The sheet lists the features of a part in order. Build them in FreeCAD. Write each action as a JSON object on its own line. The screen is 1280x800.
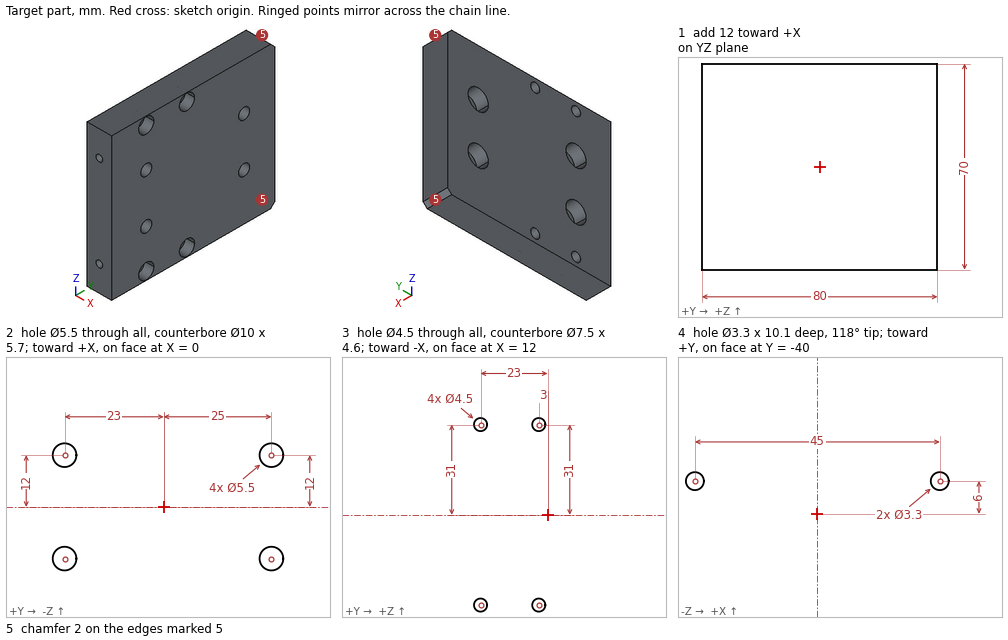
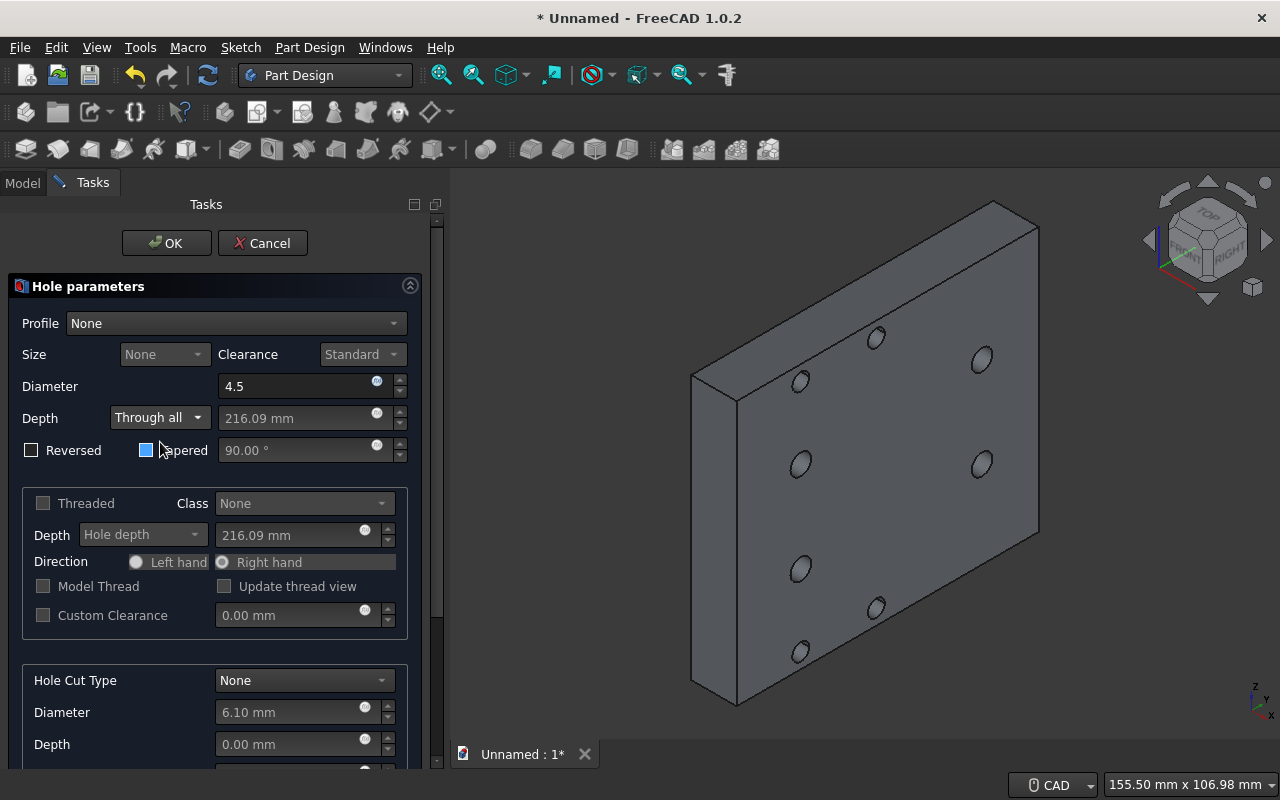
{"action": "left_click", "coordinate": [306, 680]}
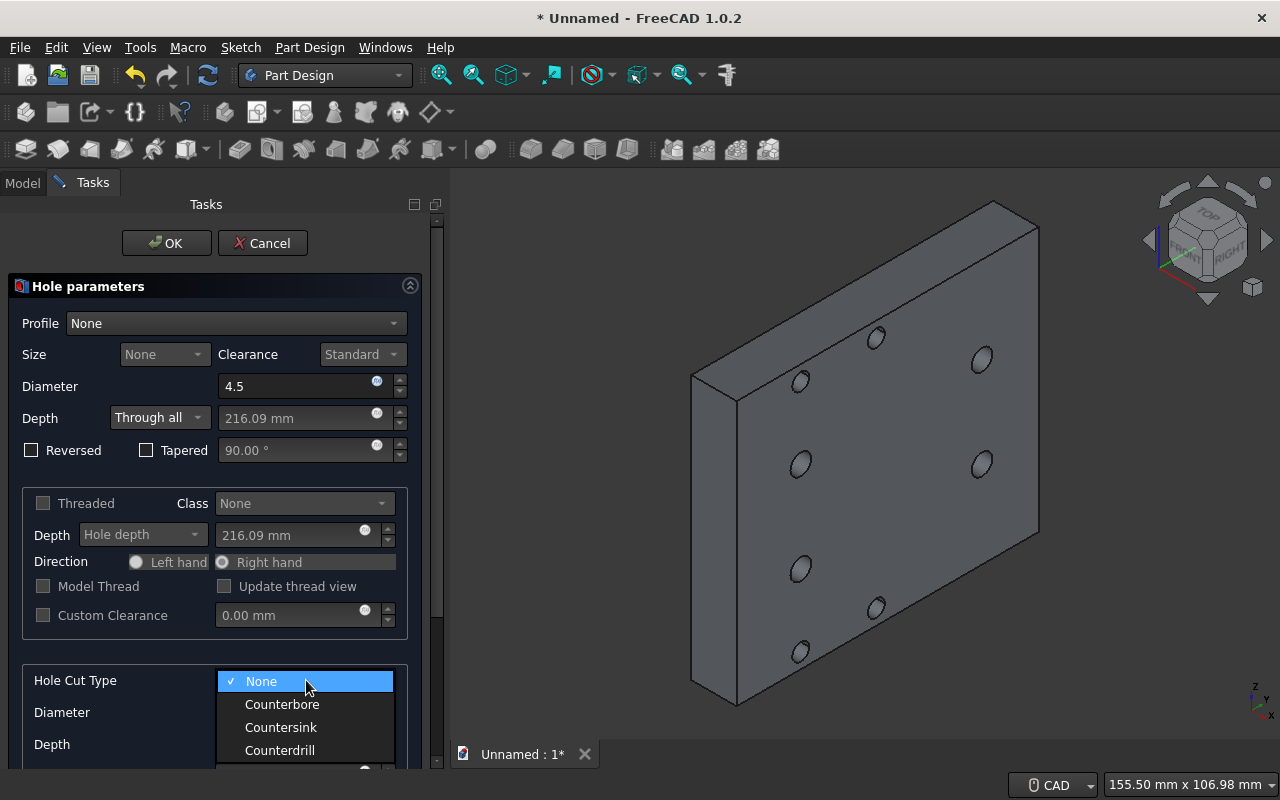
{"action": "left_click", "coordinate": [304, 704]}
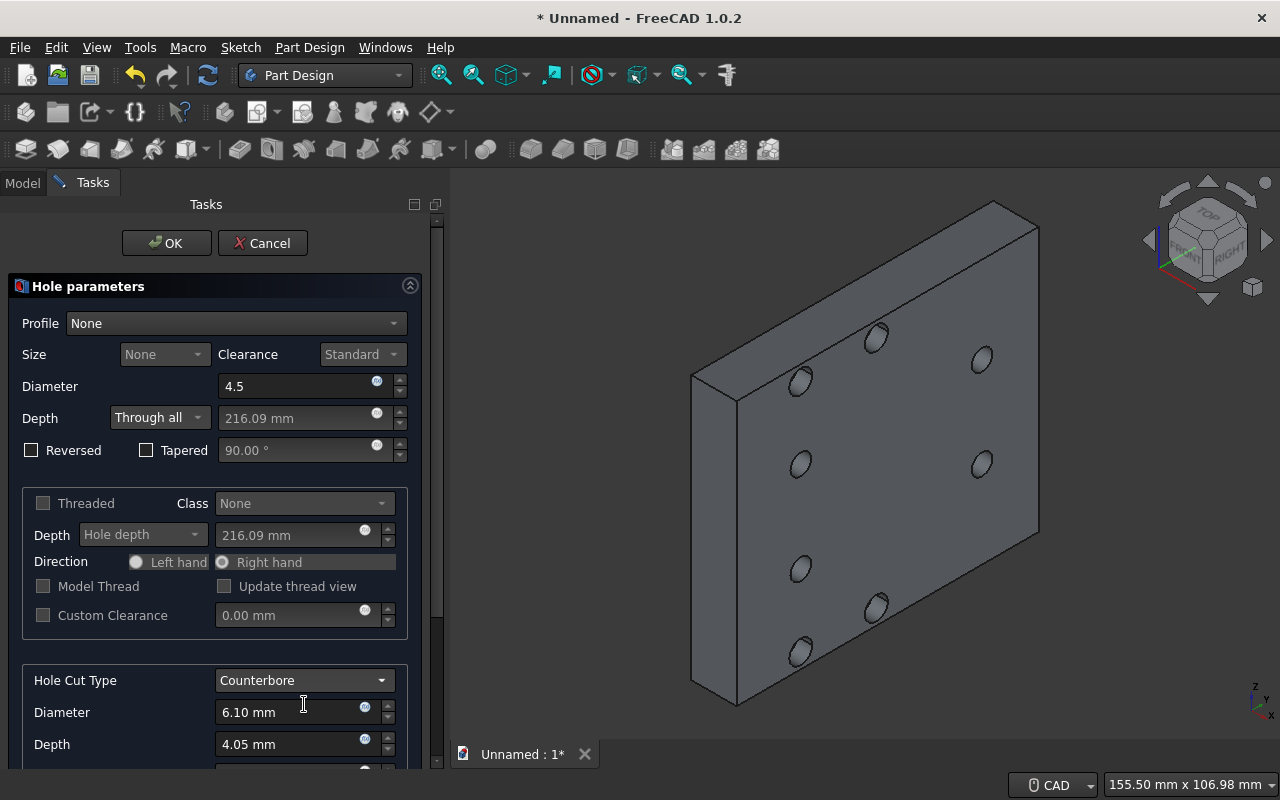
{"action": "triple_click", "coordinate": [298, 712]}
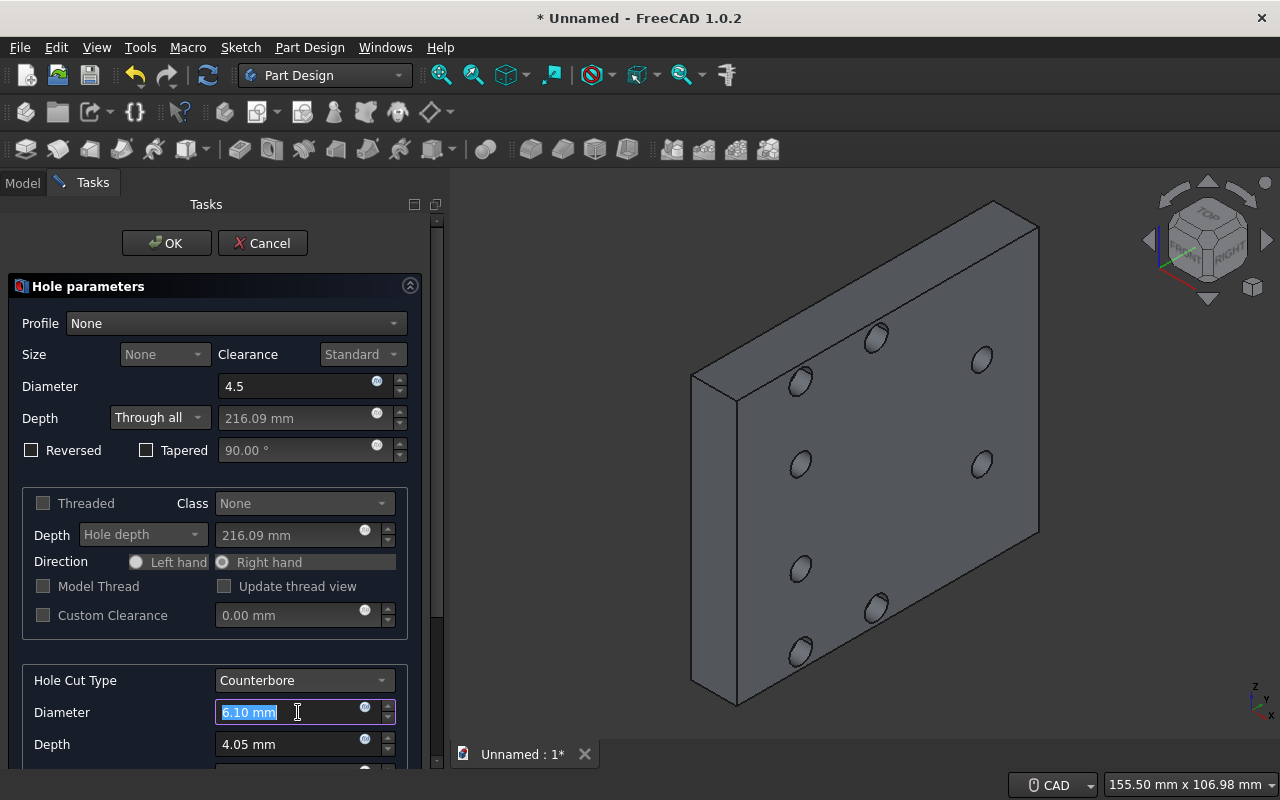
{"action": "type", "text": "7.5"}
{"action": "key", "text": "Tab"}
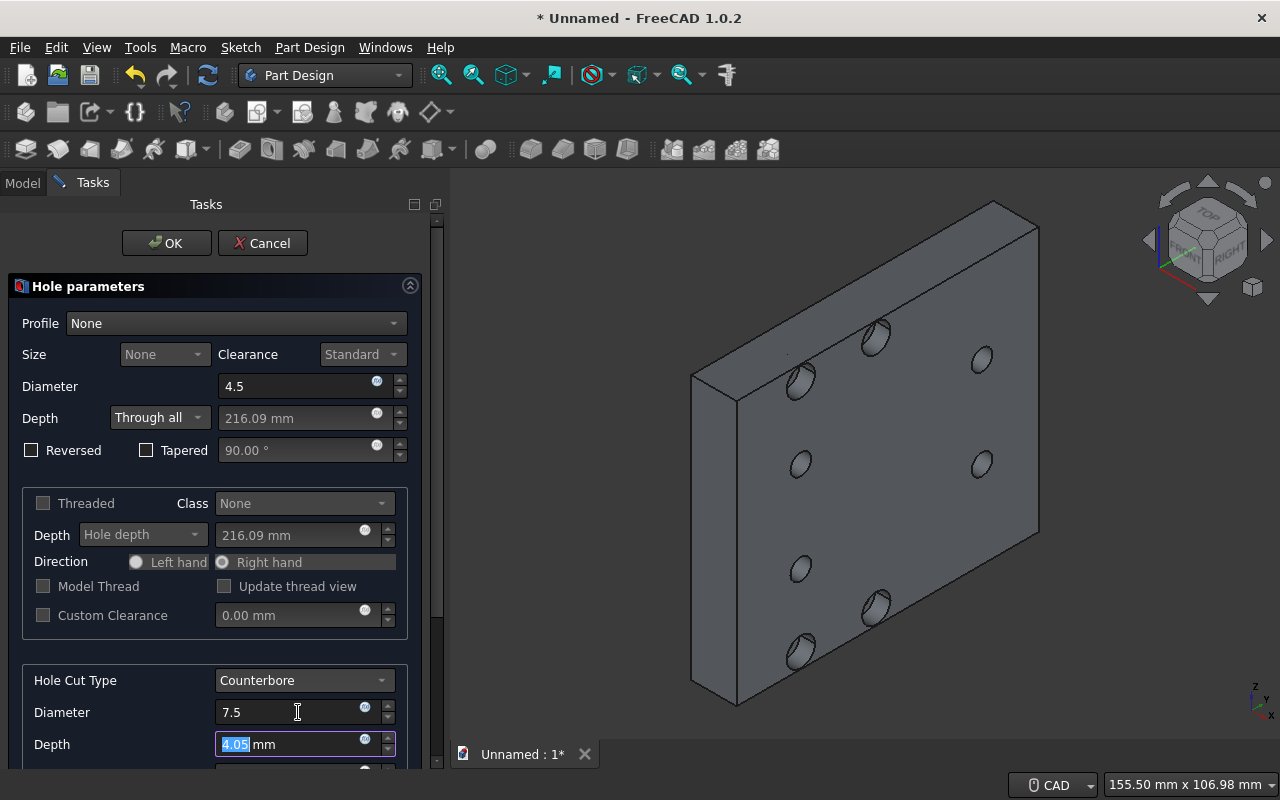
{"action": "type", "text": "4.6"}
{"action": "key", "text": "Tab"}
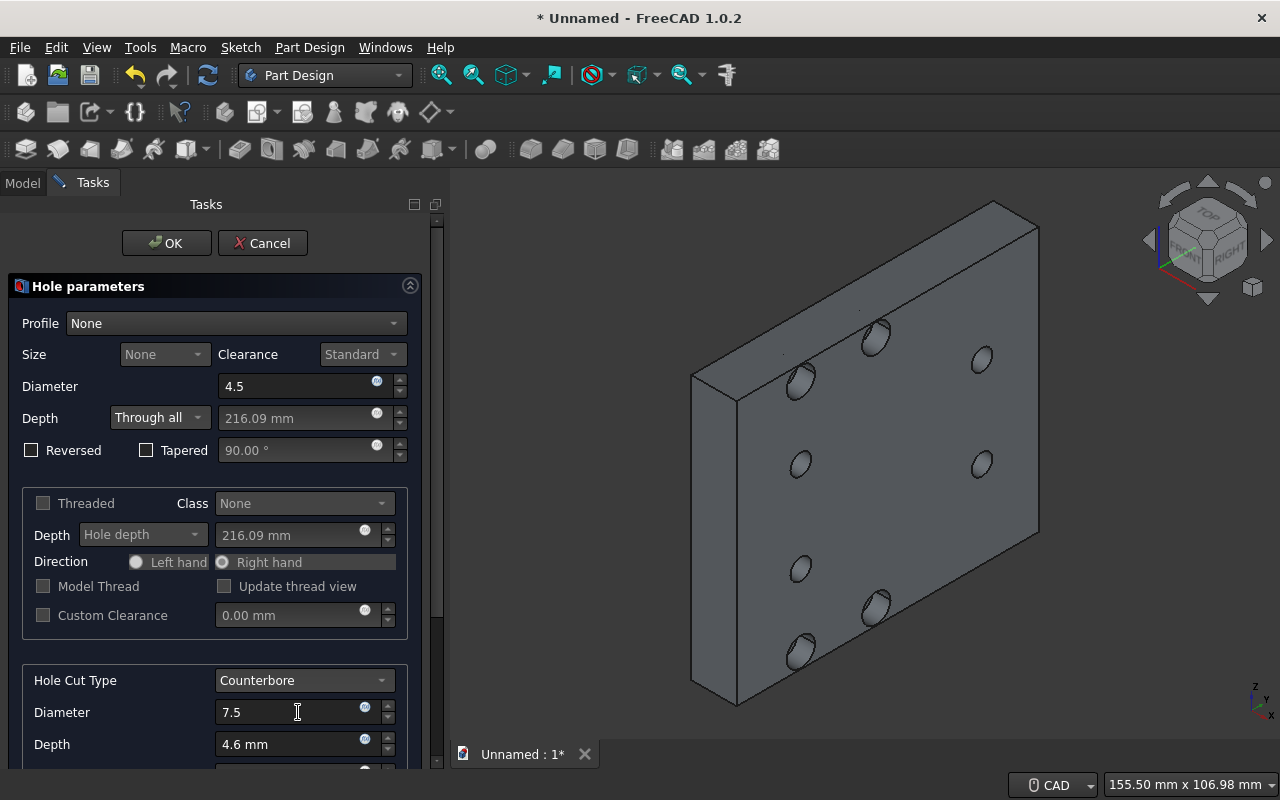
{"action": "left_click", "coordinate": [167, 243]}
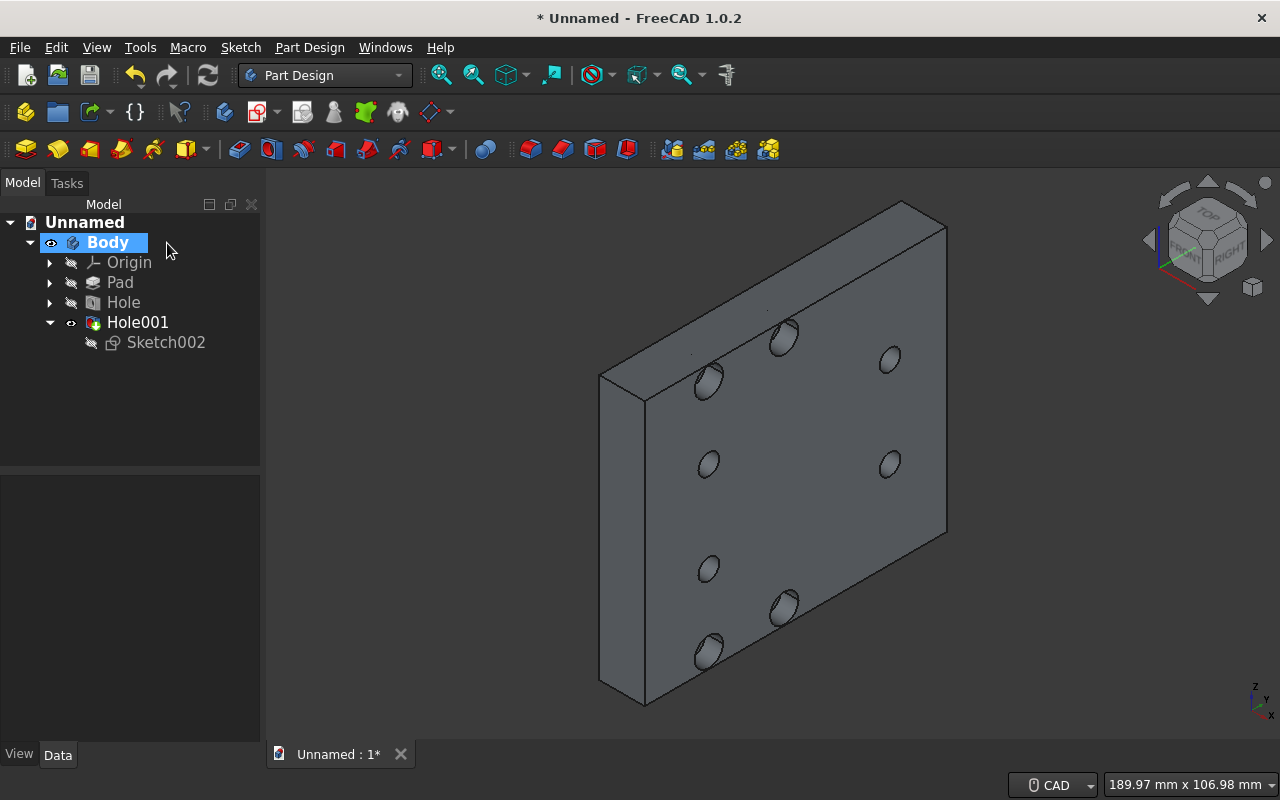
{"action": "left_click", "coordinate": [622, 627]}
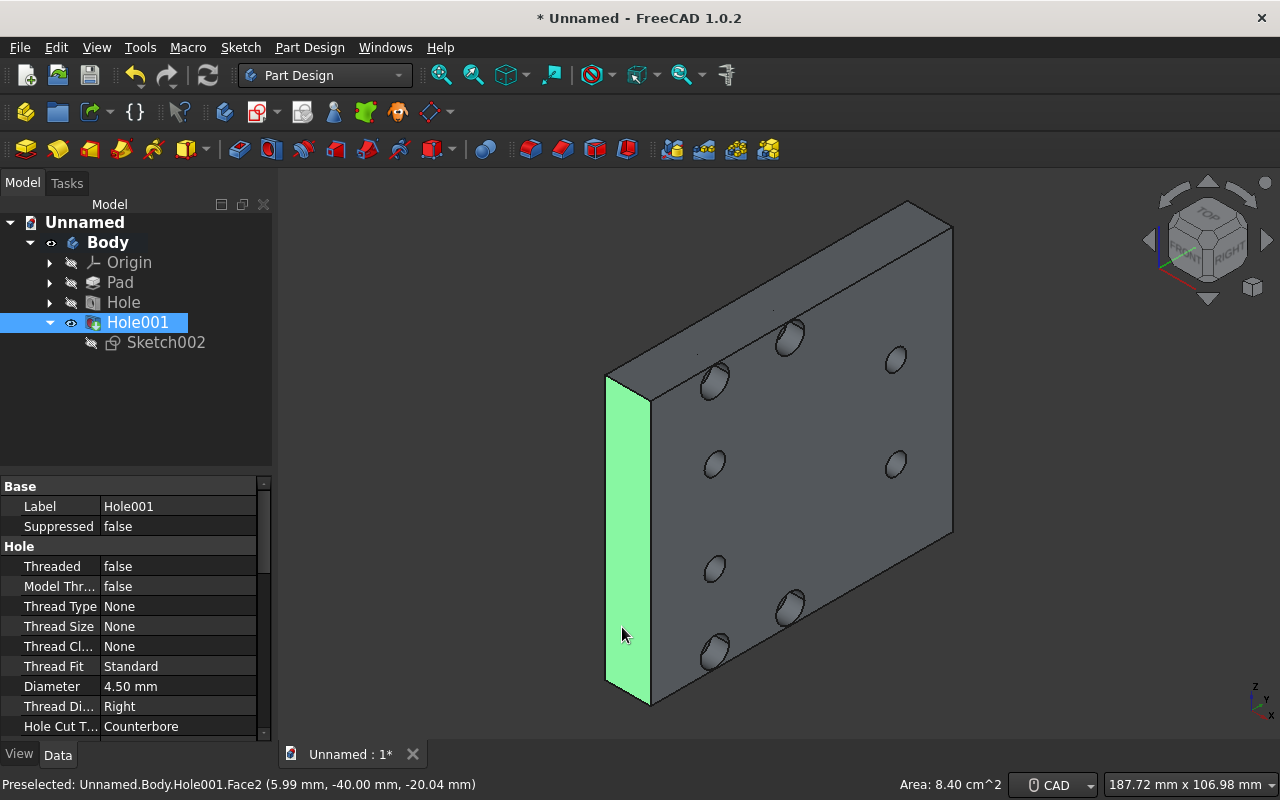
{"action": "left_click", "coordinate": [258, 112]}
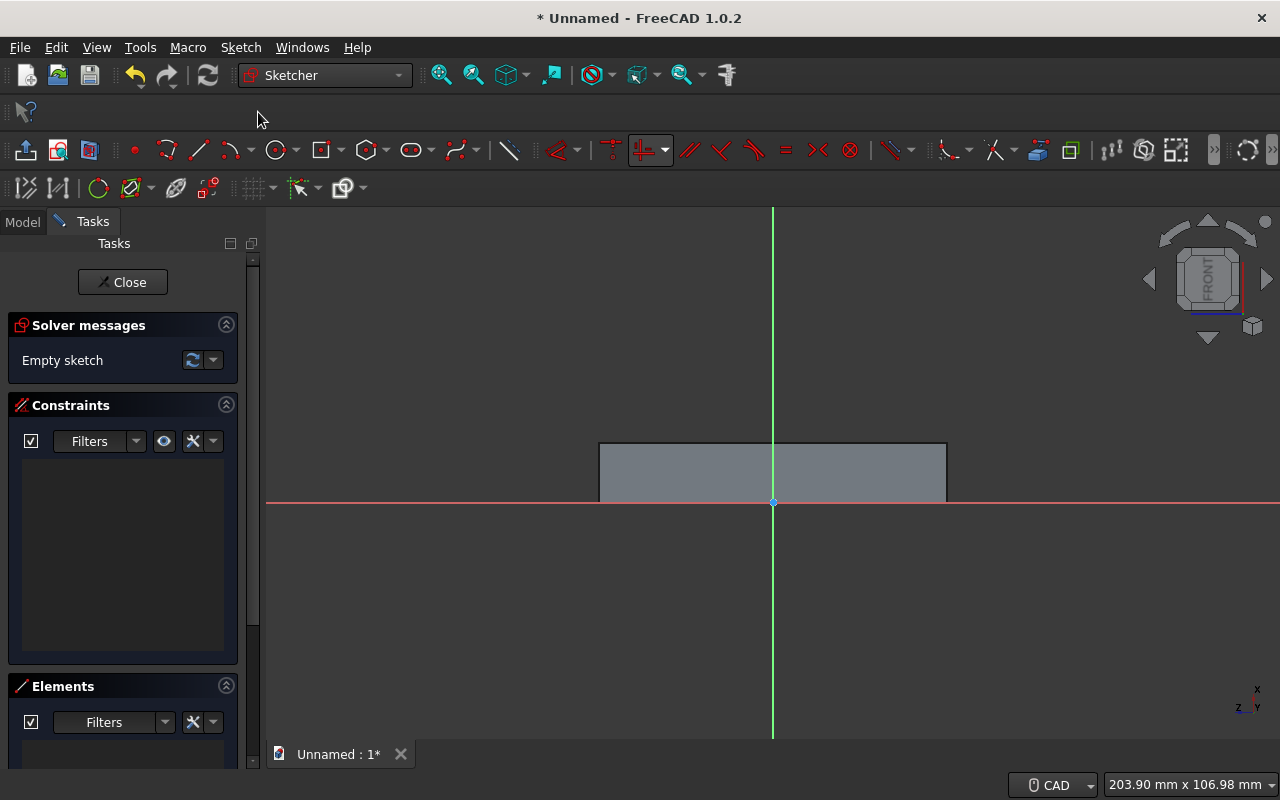
{"action": "scroll", "coordinate": [829, 493], "scroll_direction": "up", "scroll_amount": 4}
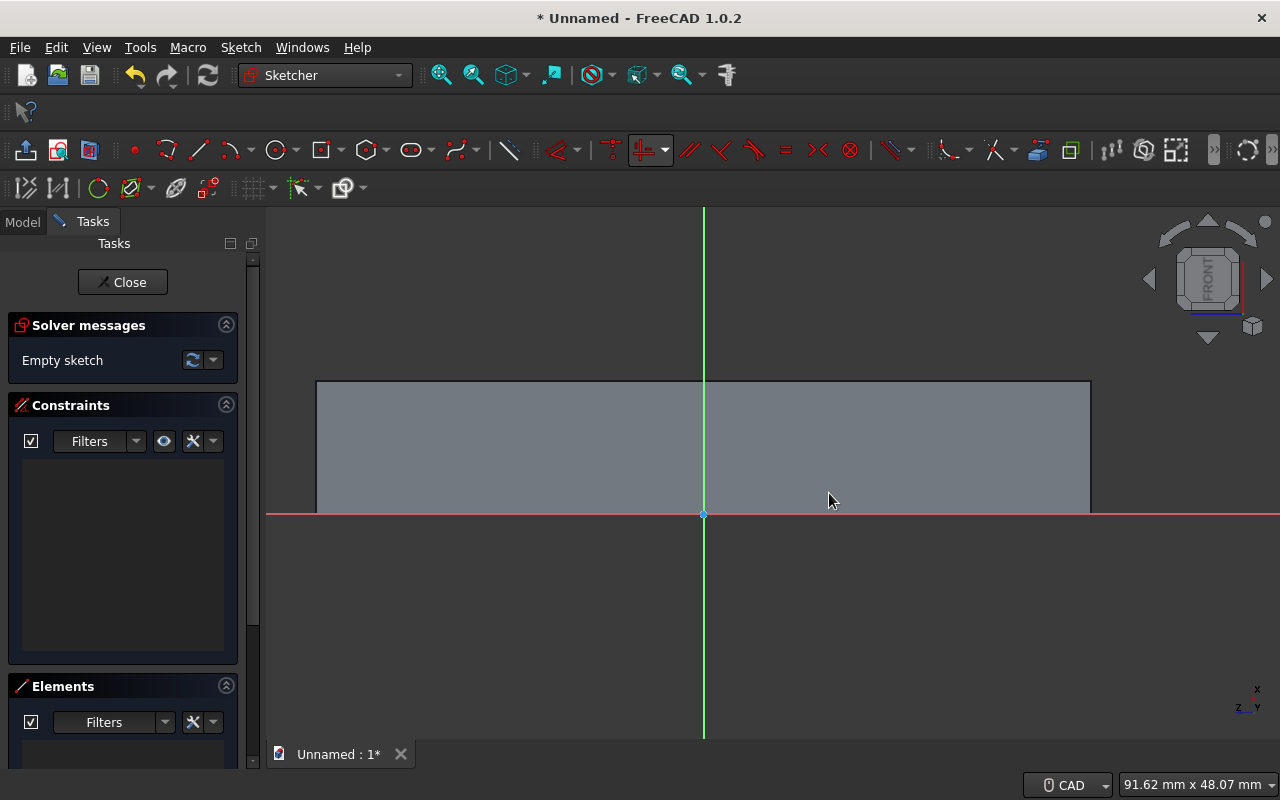
{"action": "left_click", "coordinate": [276, 150]}